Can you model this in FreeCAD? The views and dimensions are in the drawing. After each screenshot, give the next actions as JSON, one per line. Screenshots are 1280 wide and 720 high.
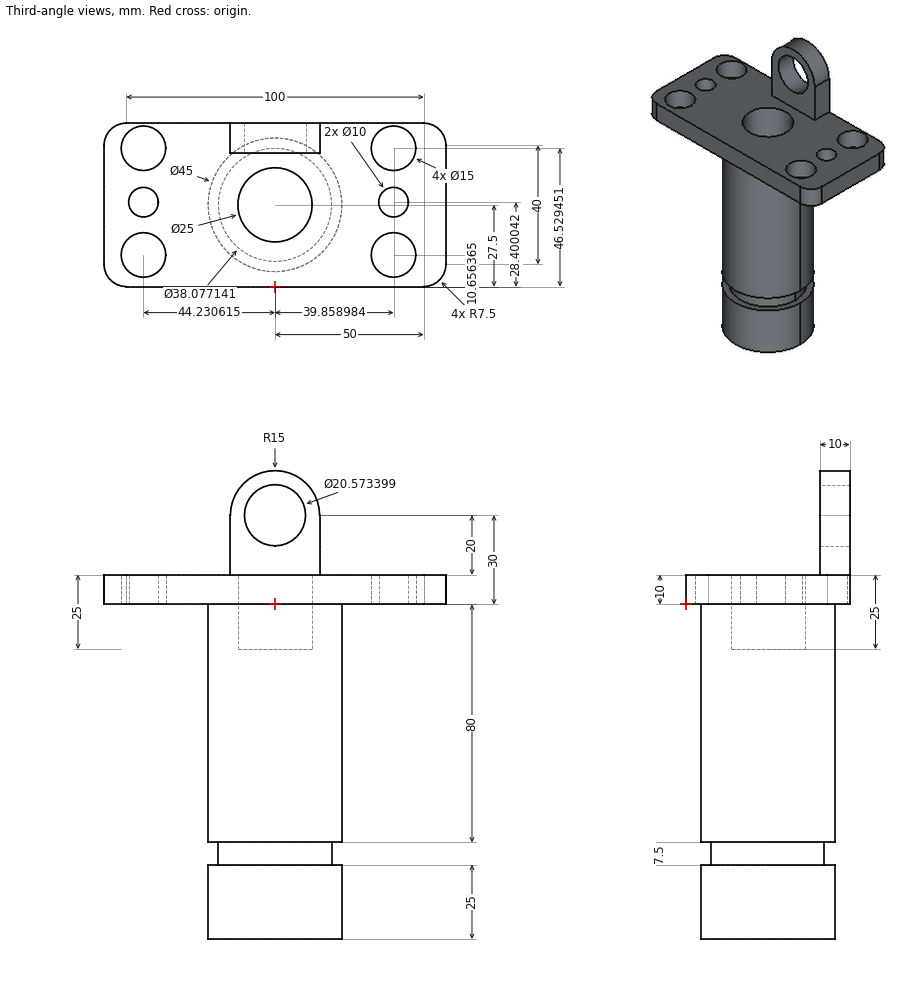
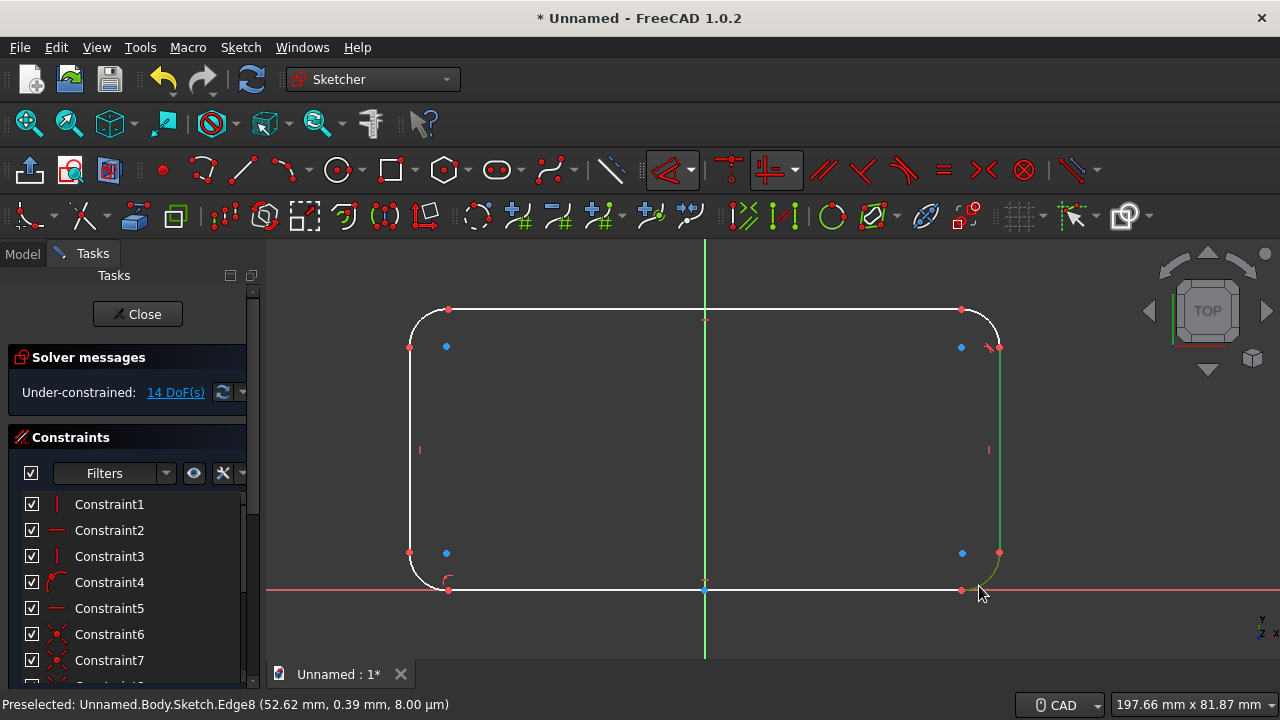
{"action": "left_click", "coordinate": [904, 170]}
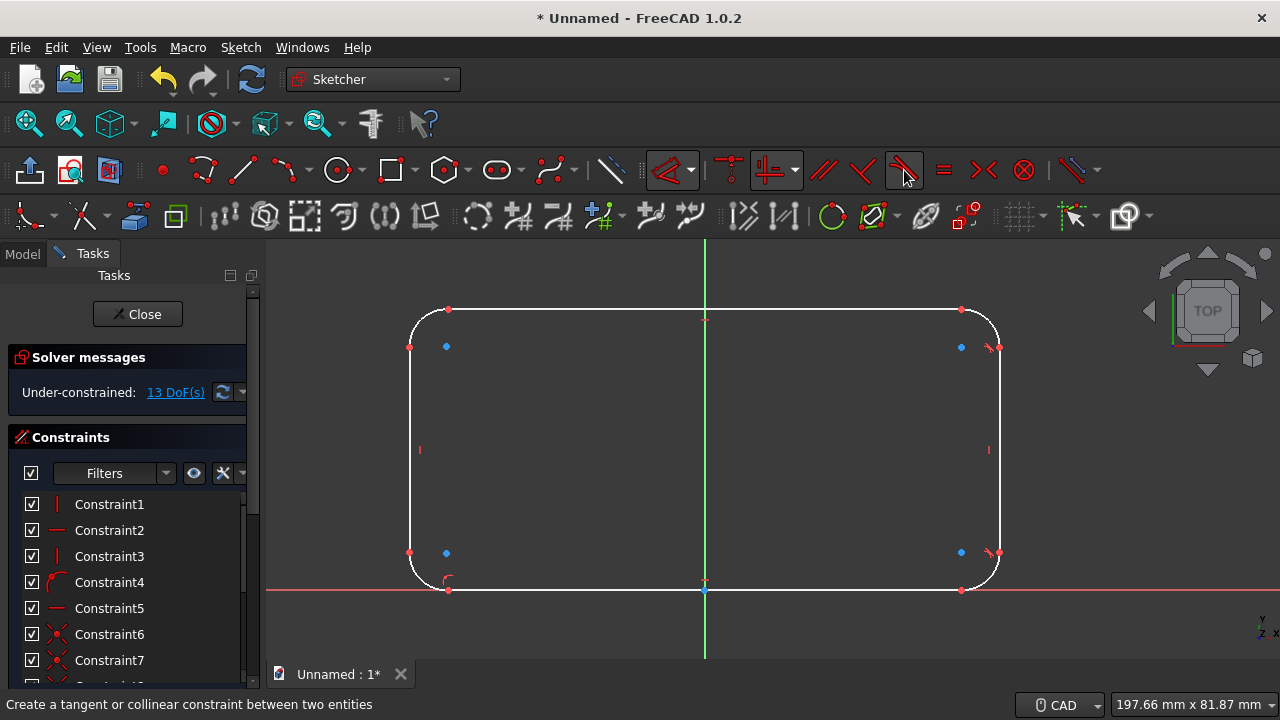
{"action": "left_click", "coordinate": [808, 309]}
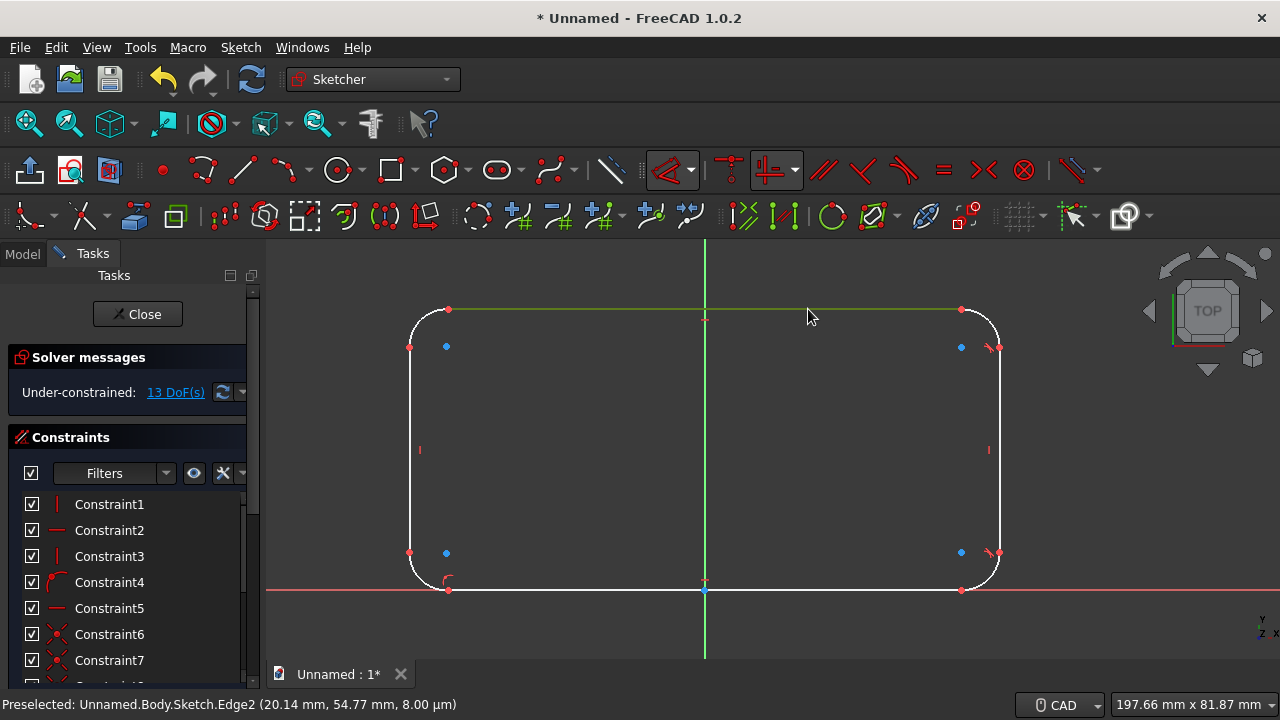
{"action": "left_click", "coordinate": [996, 330]}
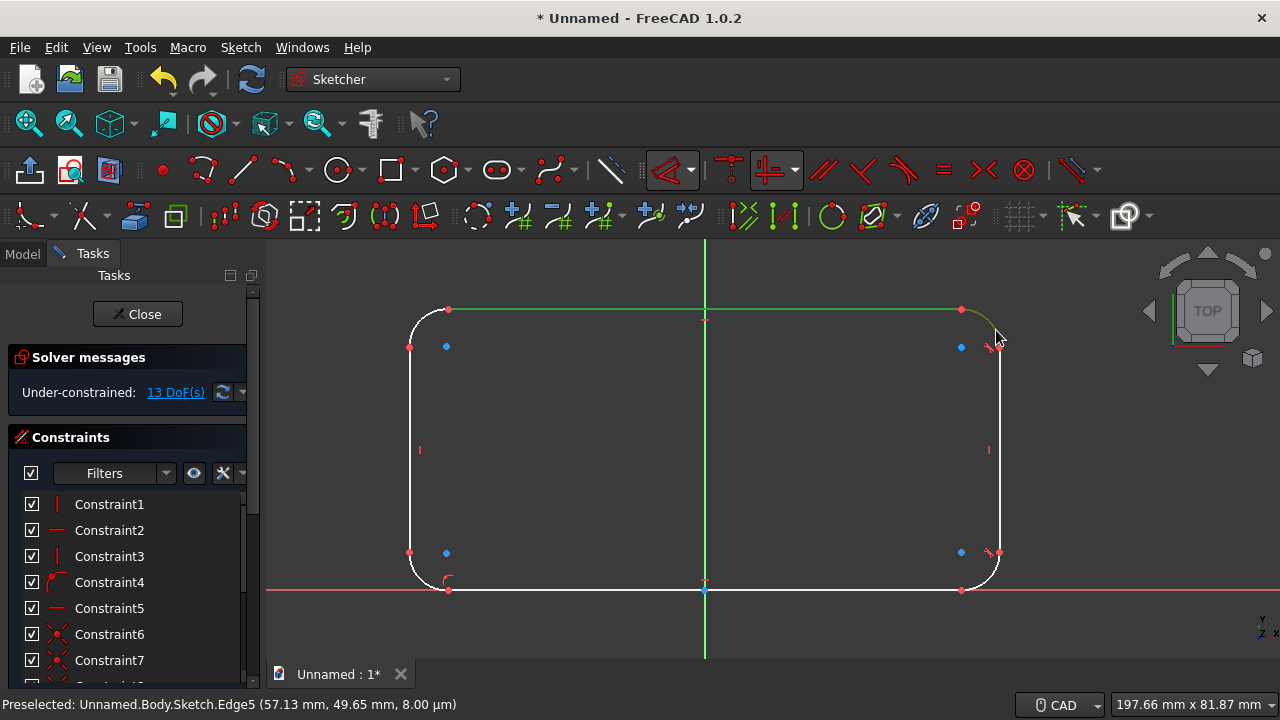
{"action": "left_click", "coordinate": [904, 170]}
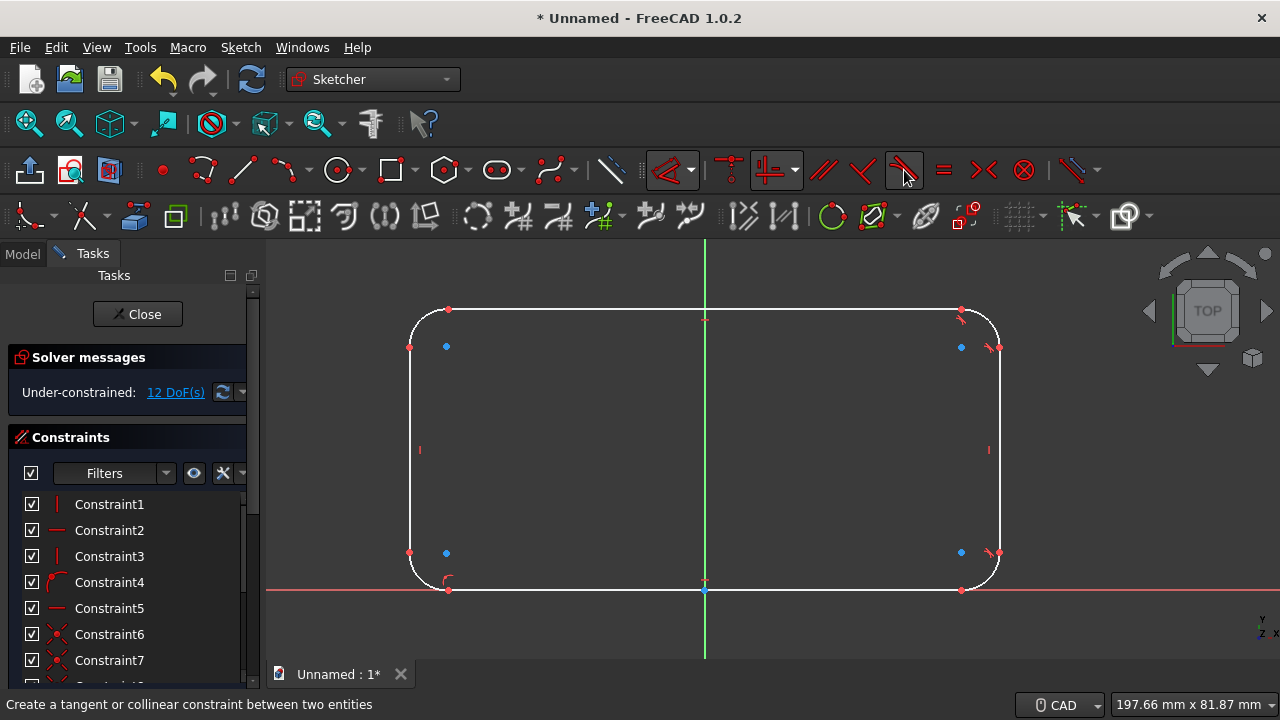
{"action": "left_click", "coordinate": [808, 309]}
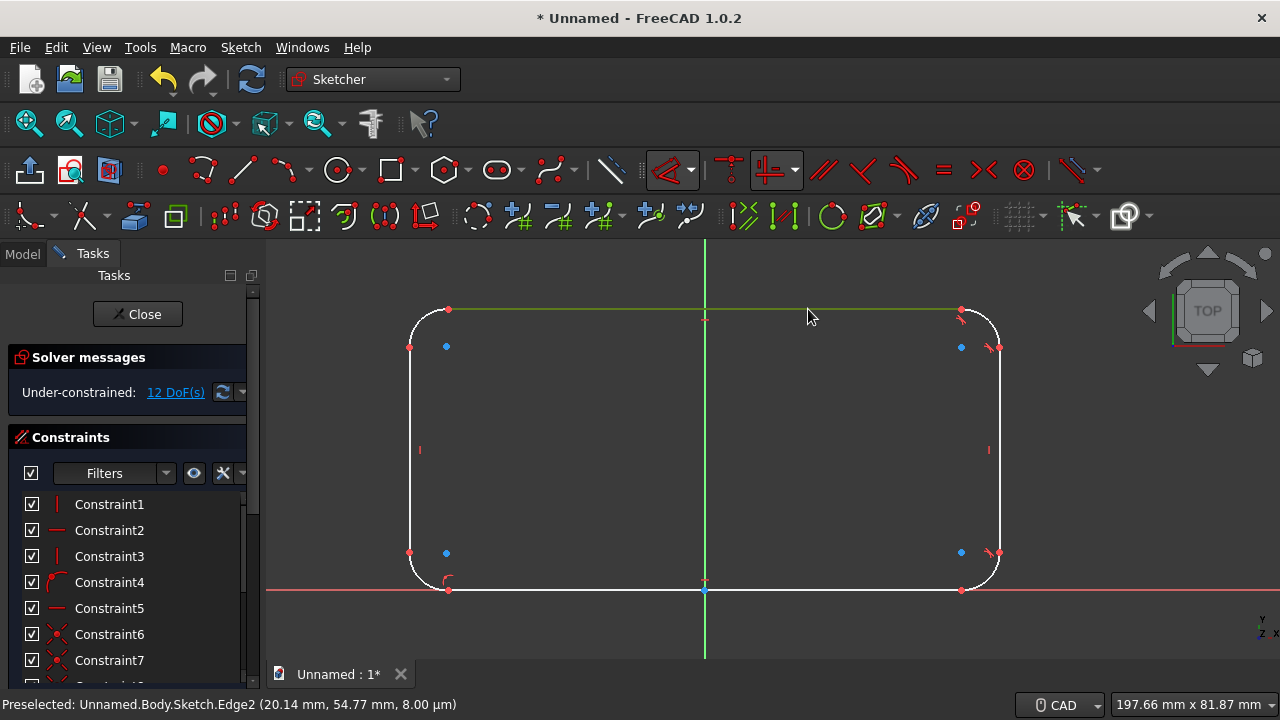
{"action": "left_click", "coordinate": [431, 313]}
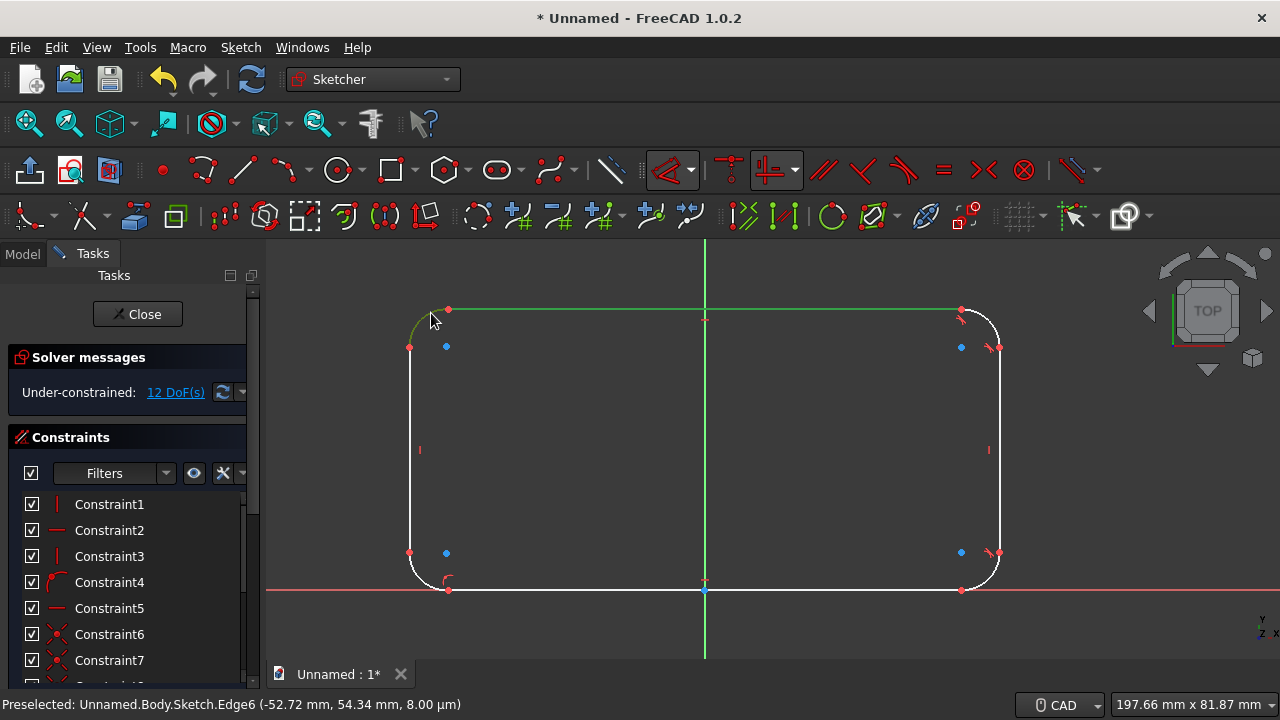
{"action": "key", "text": "t"}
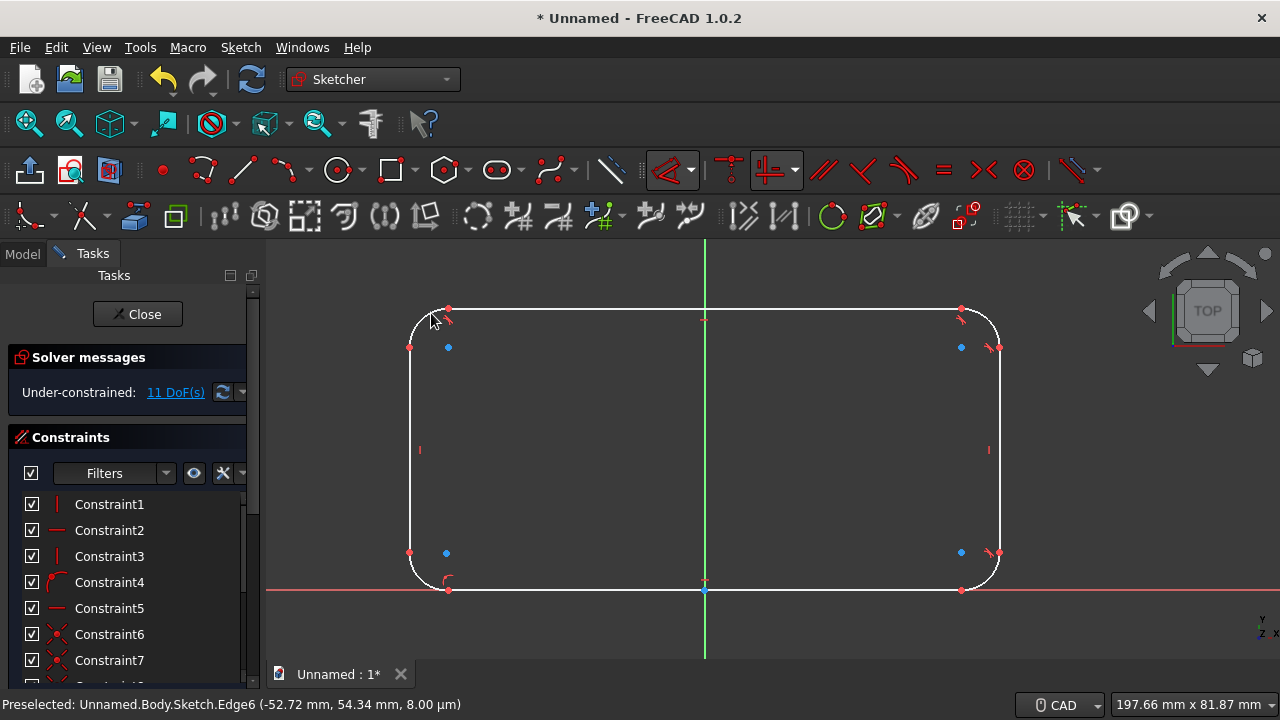
{"action": "left_click", "coordinate": [410, 409]}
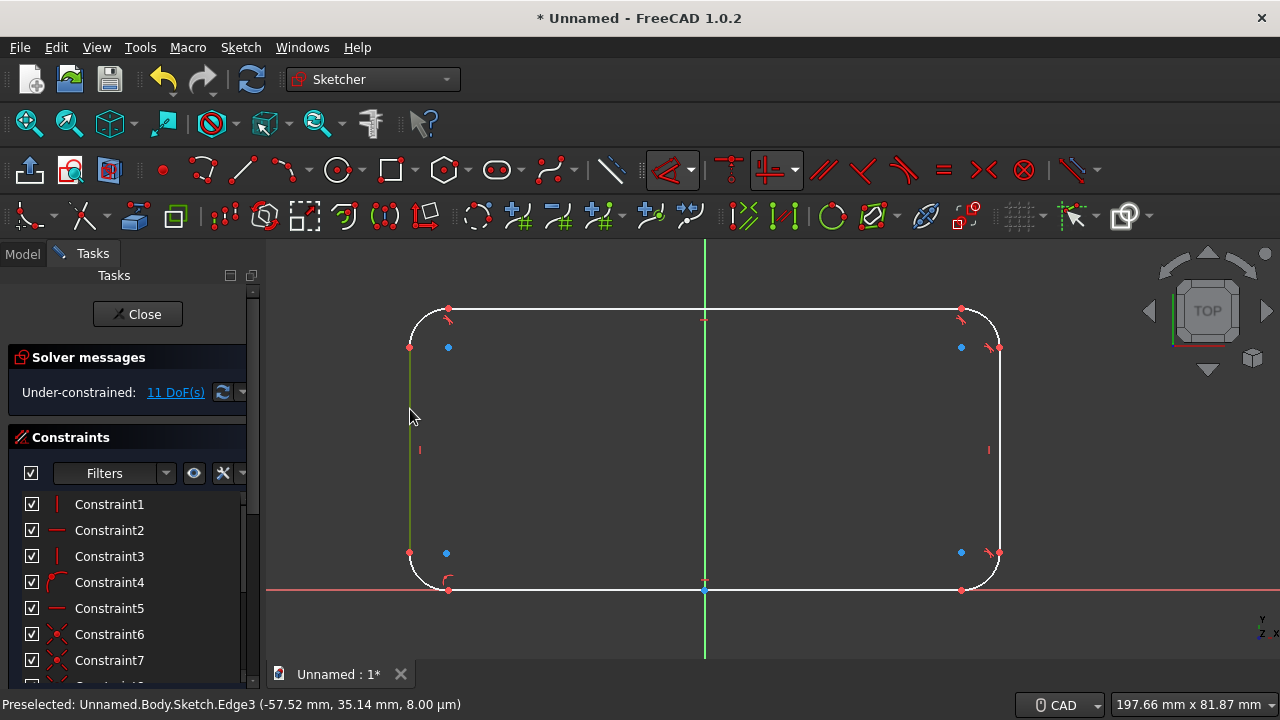
{"action": "left_click", "coordinate": [431, 313]}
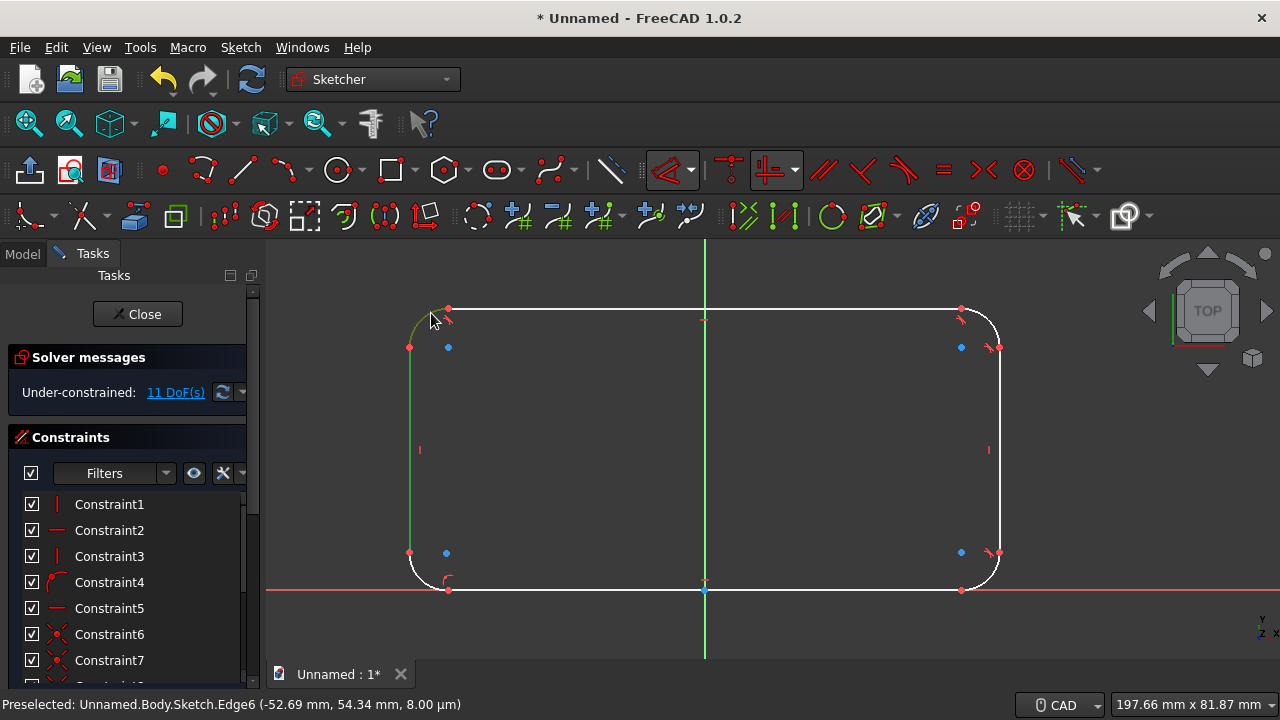
{"action": "key", "text": "t"}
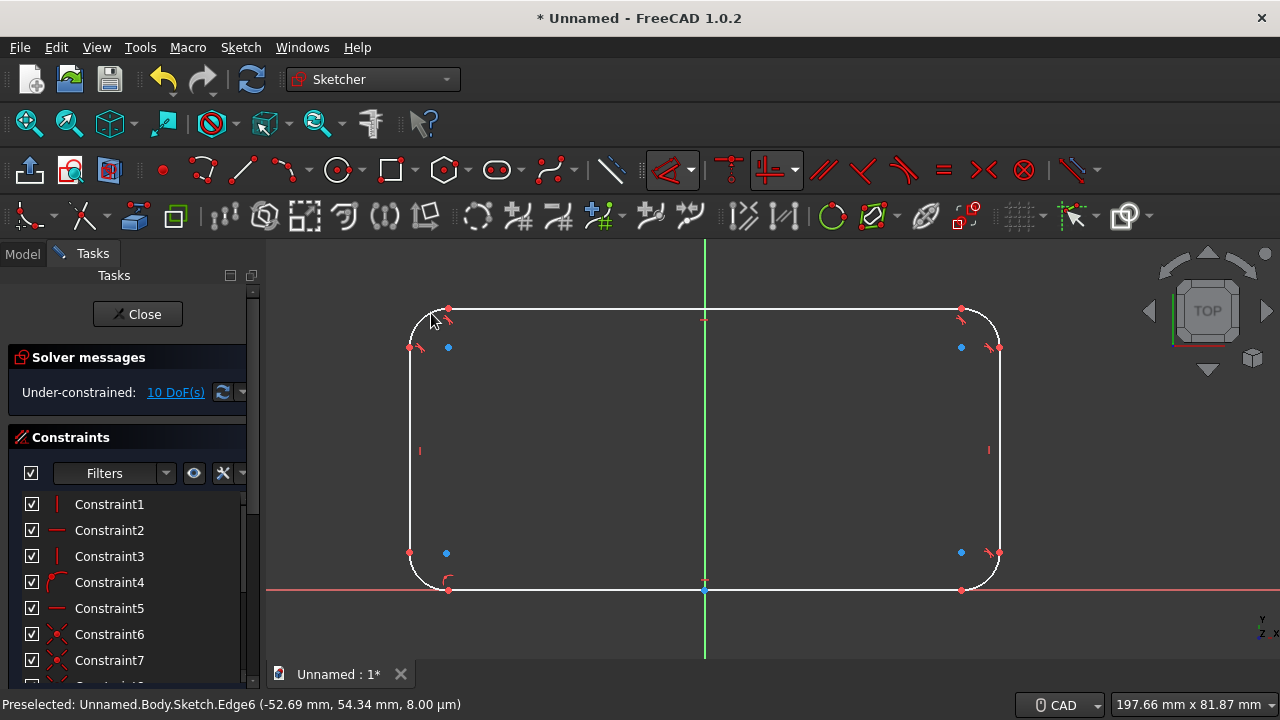
{"action": "left_click", "coordinate": [410, 409]}